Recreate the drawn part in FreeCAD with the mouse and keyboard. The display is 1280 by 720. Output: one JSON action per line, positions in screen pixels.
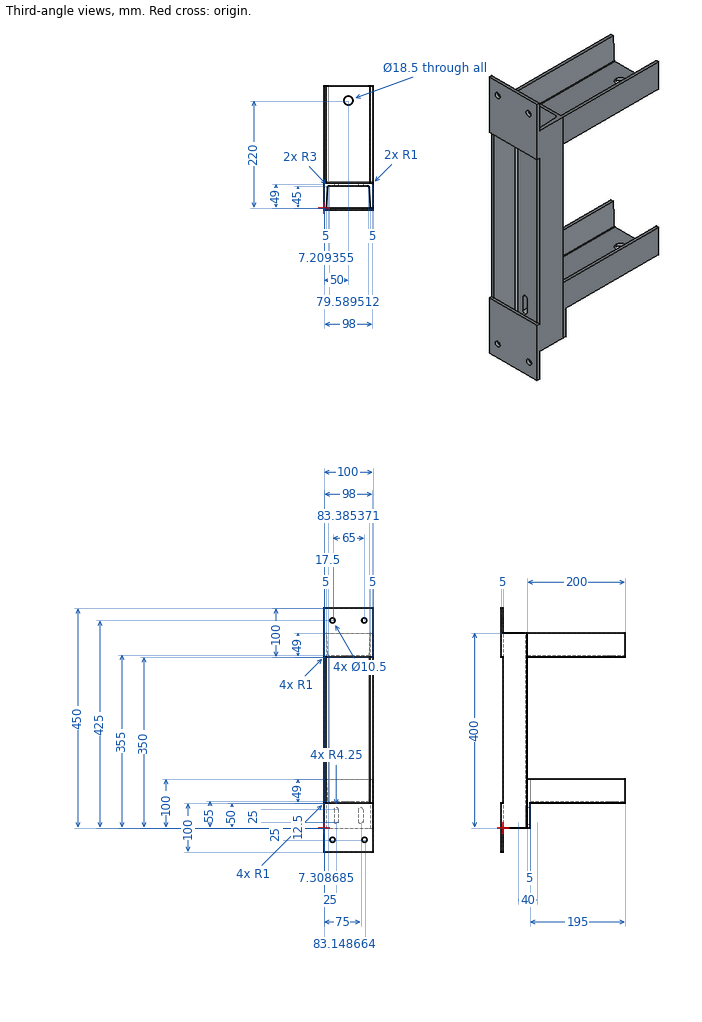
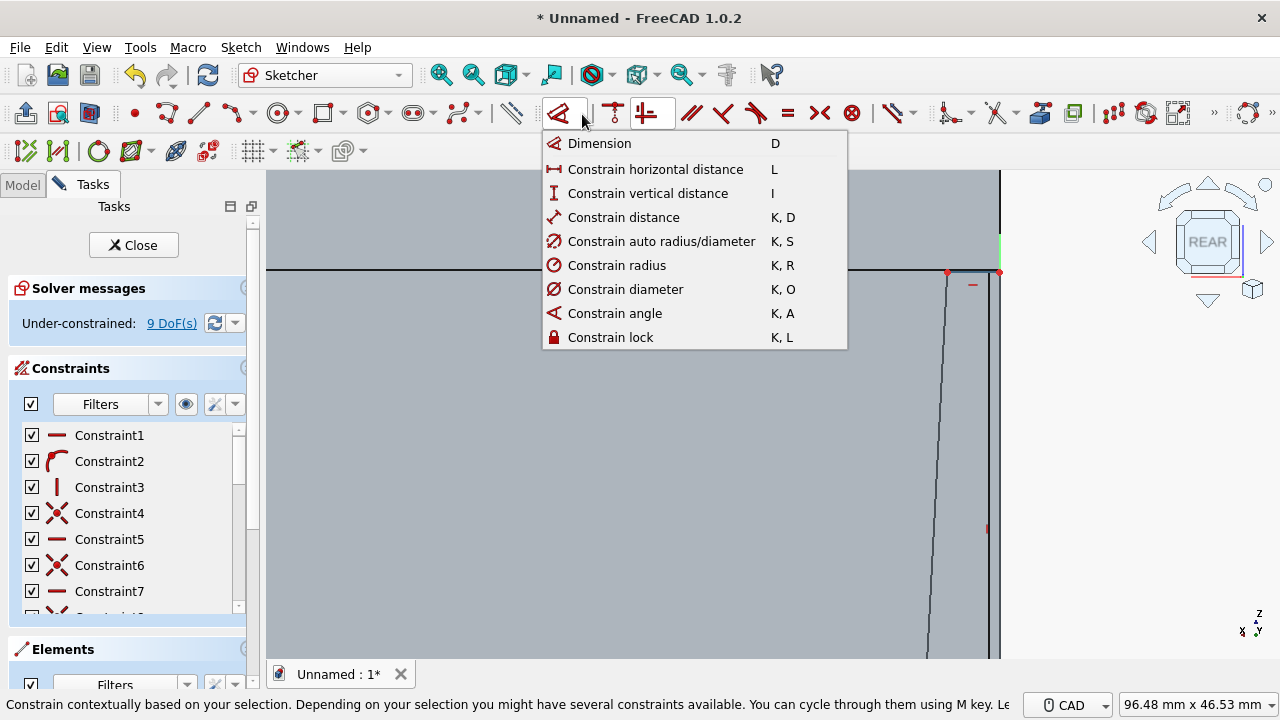
{"action": "left_click", "coordinate": [695, 169]}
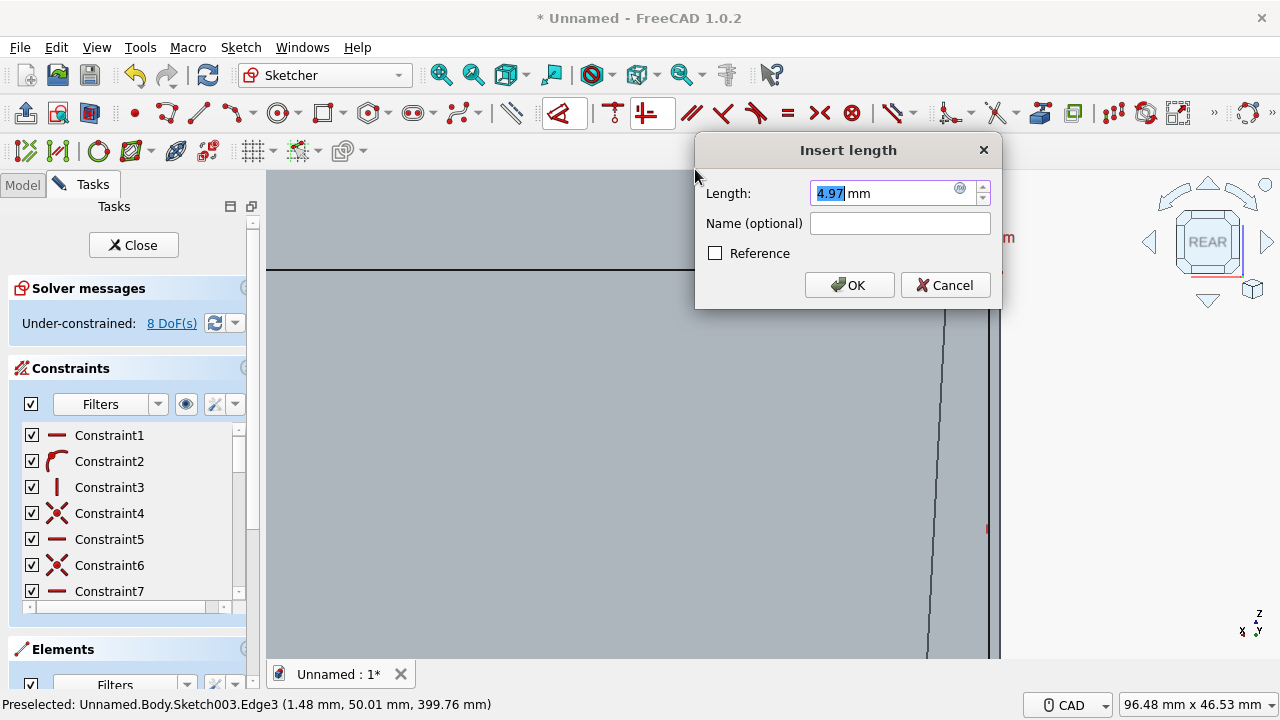
{"action": "type", "text": "5"}
{"action": "key", "text": "Return"}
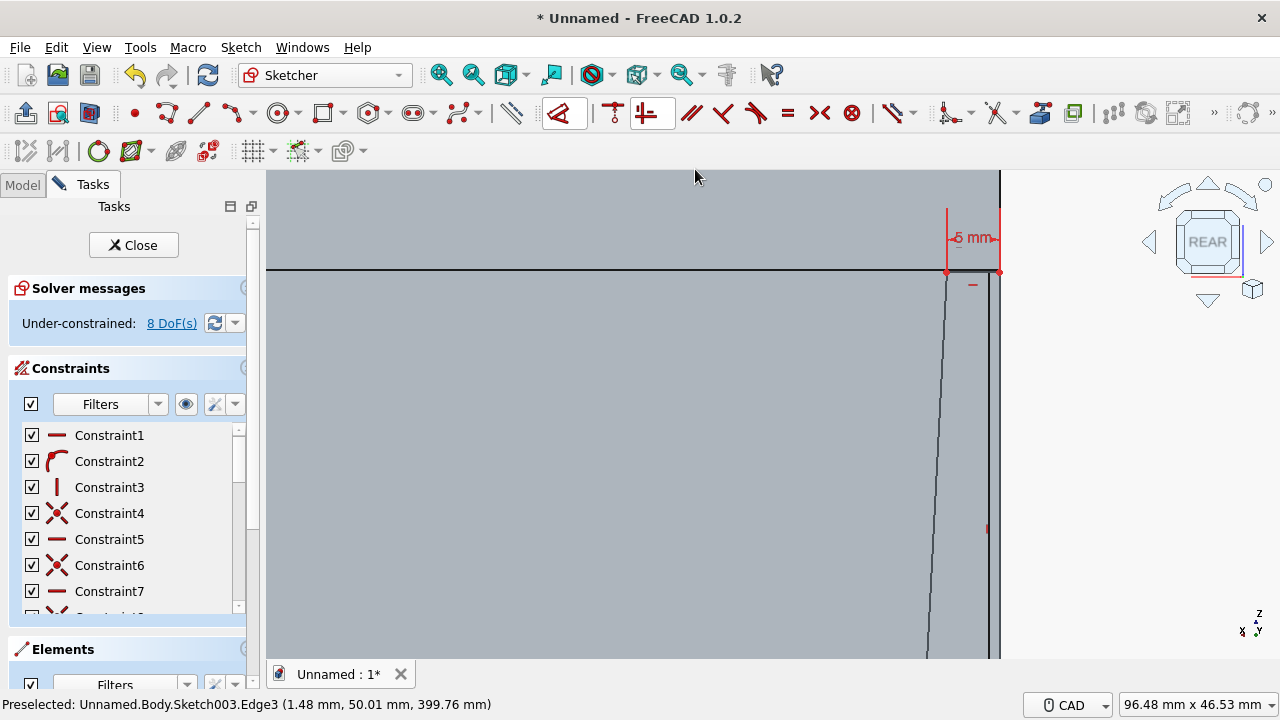
{"action": "scroll", "coordinate": [985, 271], "scroll_direction": "down", "scroll_amount": 3}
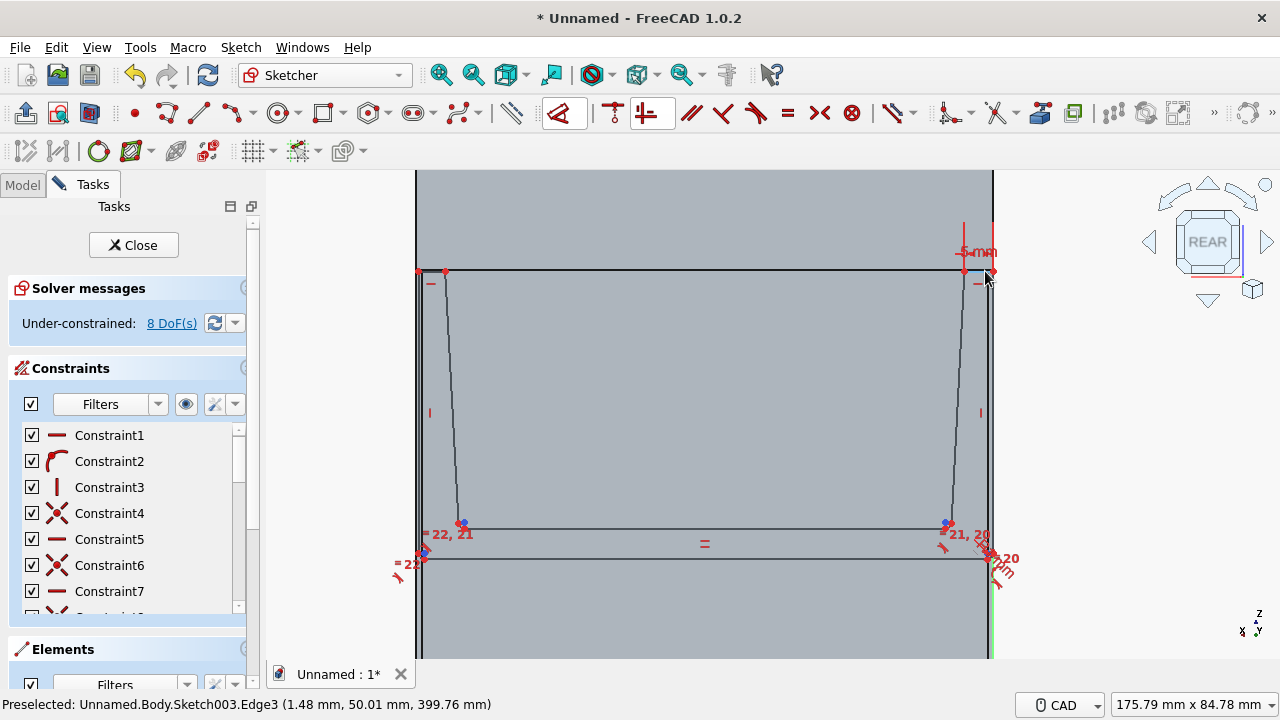
{"action": "scroll", "coordinate": [437, 272], "scroll_direction": "up", "scroll_amount": 3}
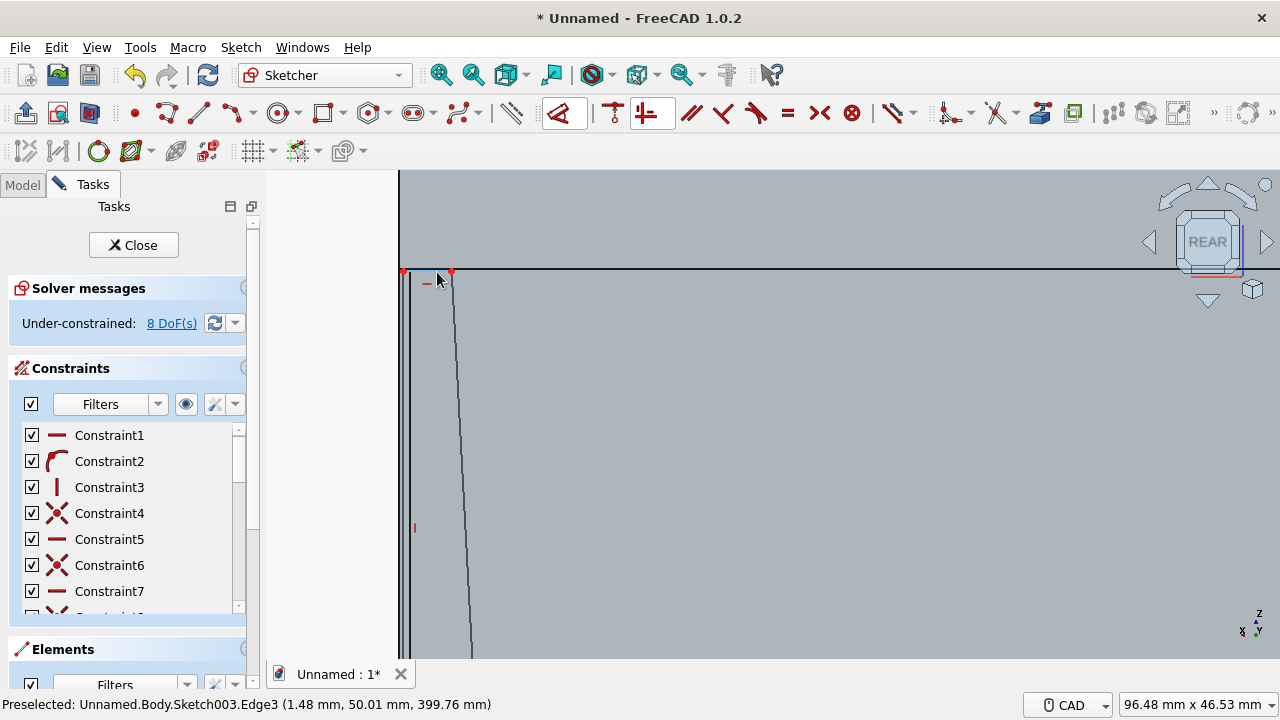
{"action": "left_click", "coordinate": [437, 271]}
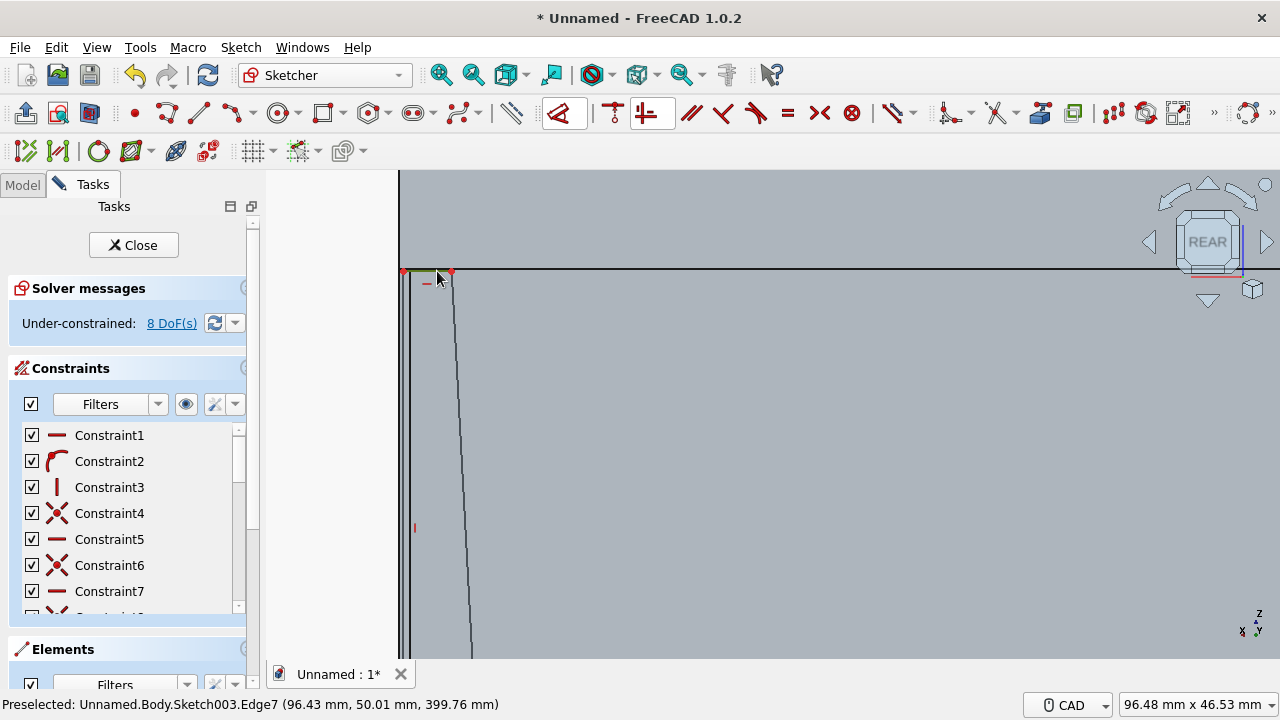
{"action": "key", "text": "l"}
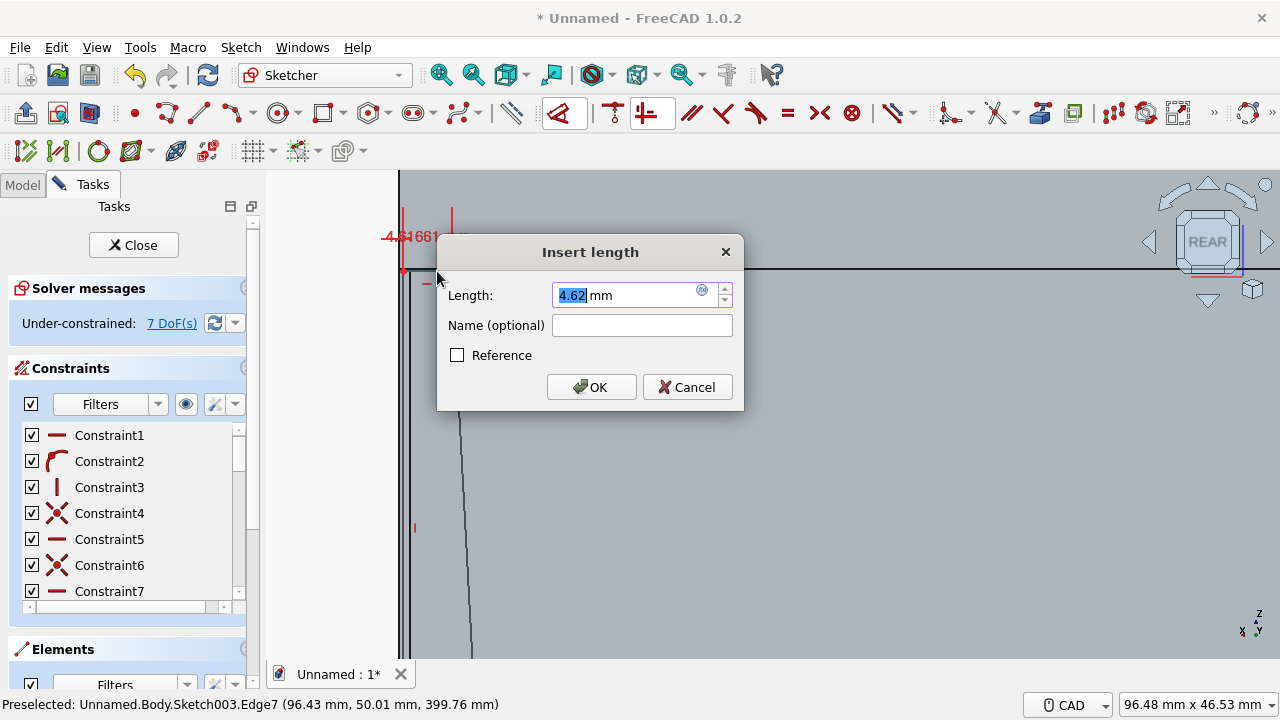
{"action": "type", "text": "5"}
{"action": "key", "text": "Return"}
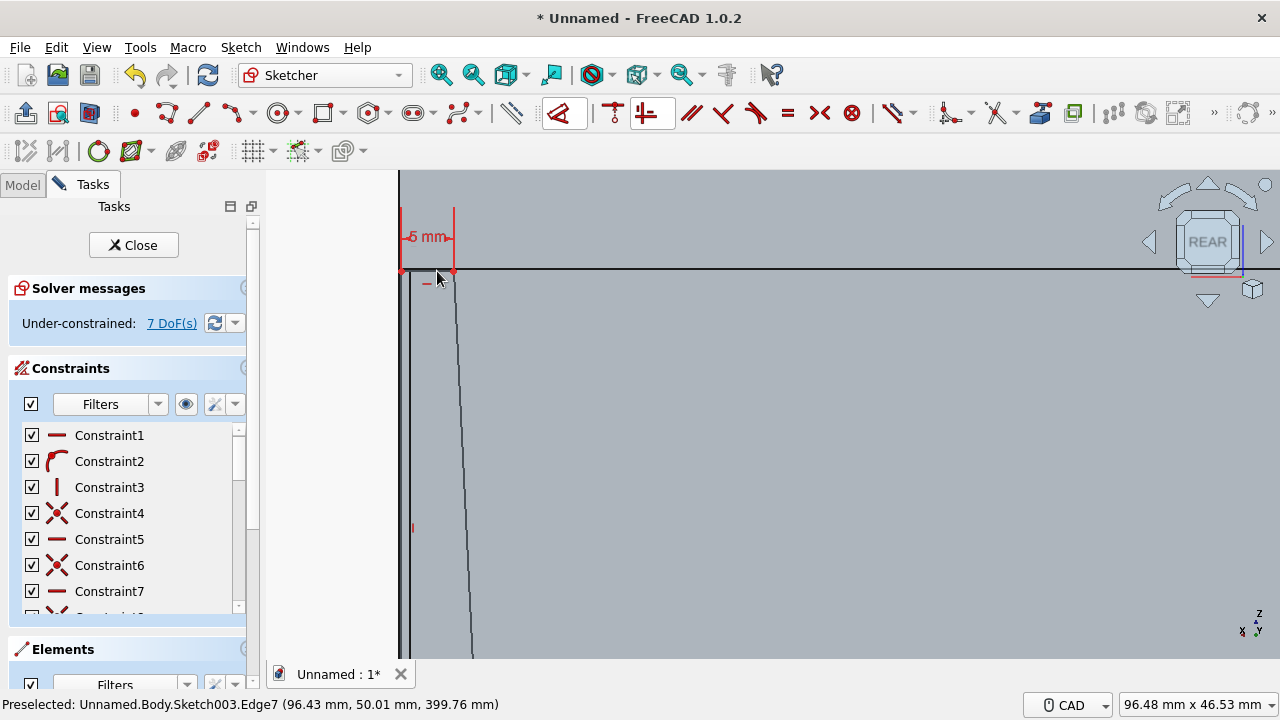
{"action": "scroll", "coordinate": [436, 272], "scroll_direction": "down", "scroll_amount": 3}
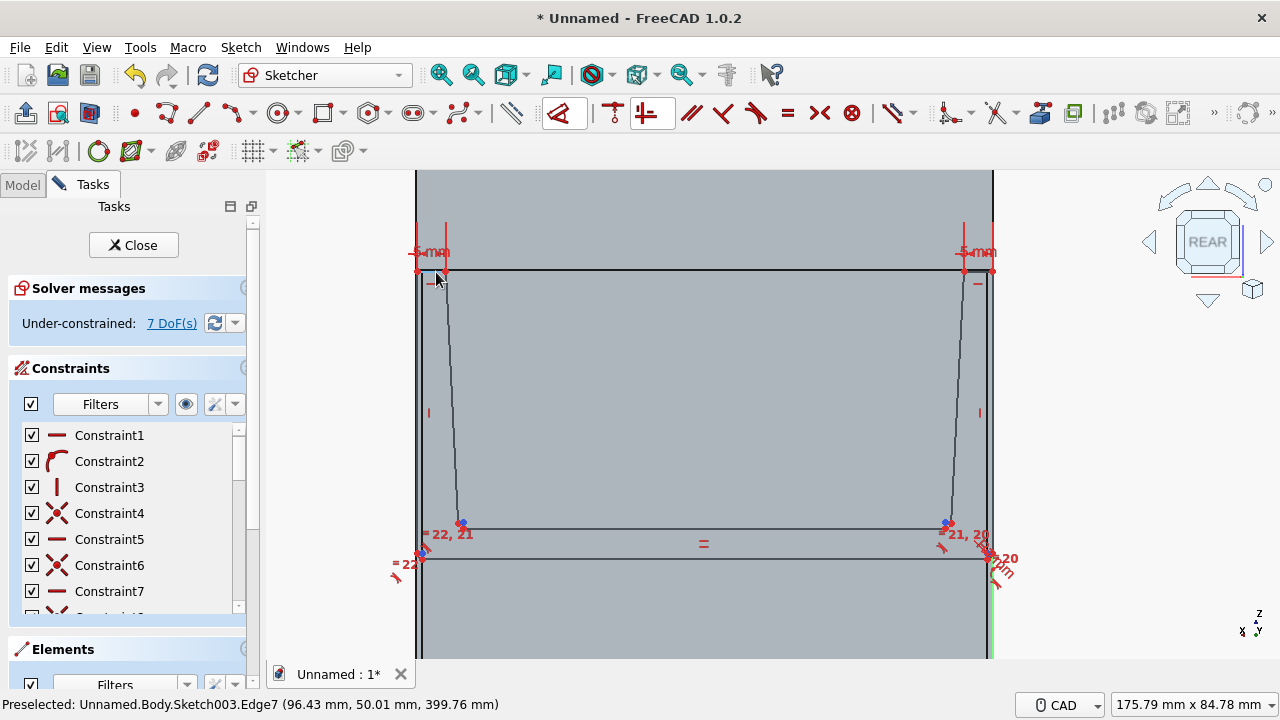
{"action": "left_click", "coordinate": [592, 559]}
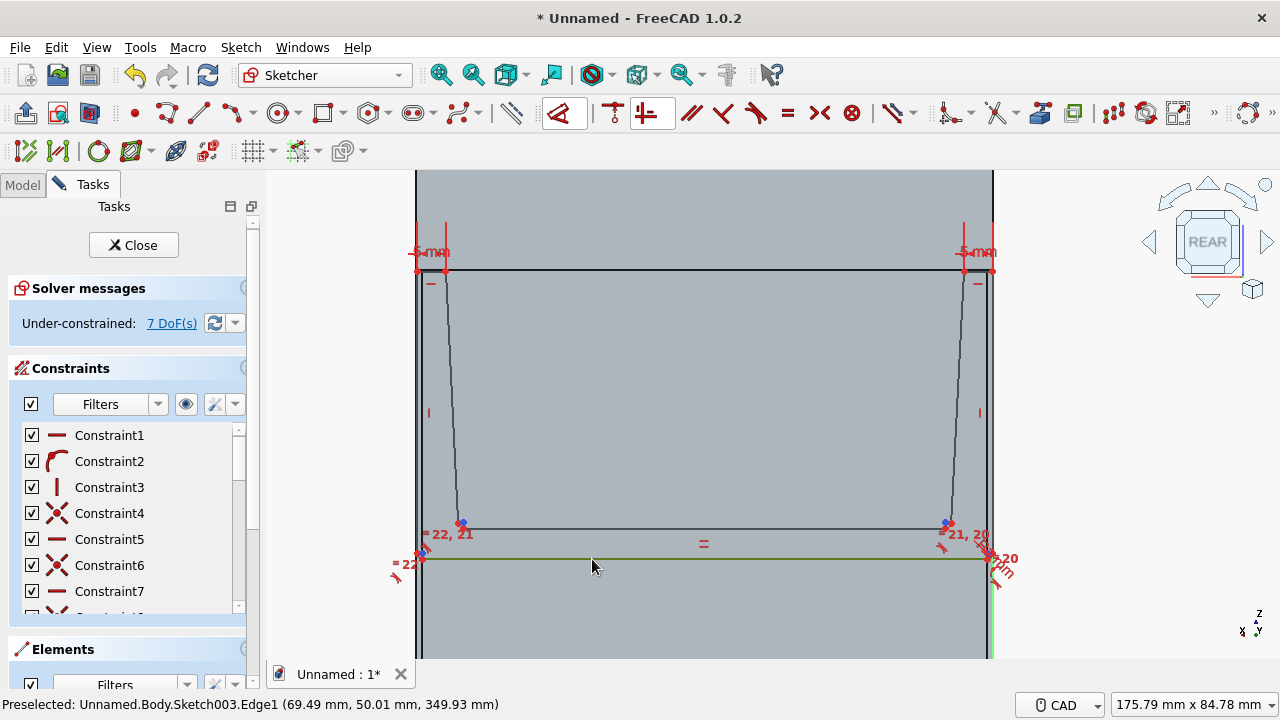
{"action": "left_click", "coordinate": [582, 114]}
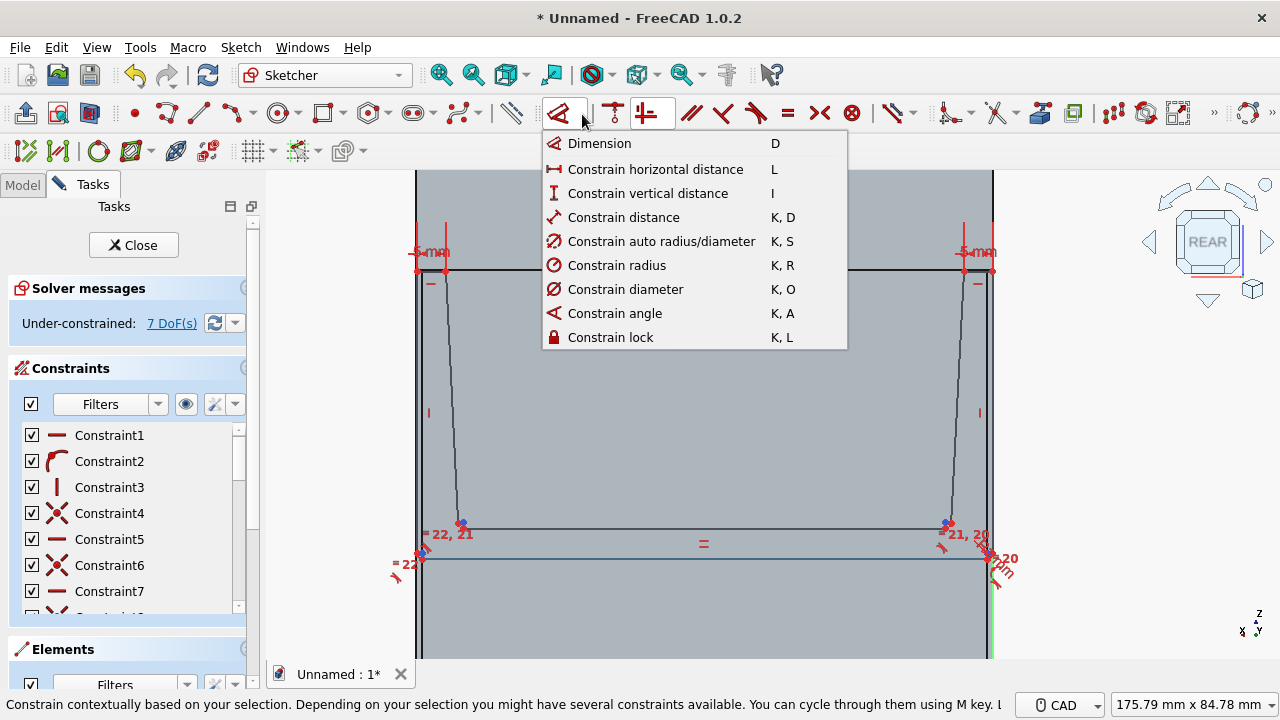
{"action": "left_click", "coordinate": [695, 169]}